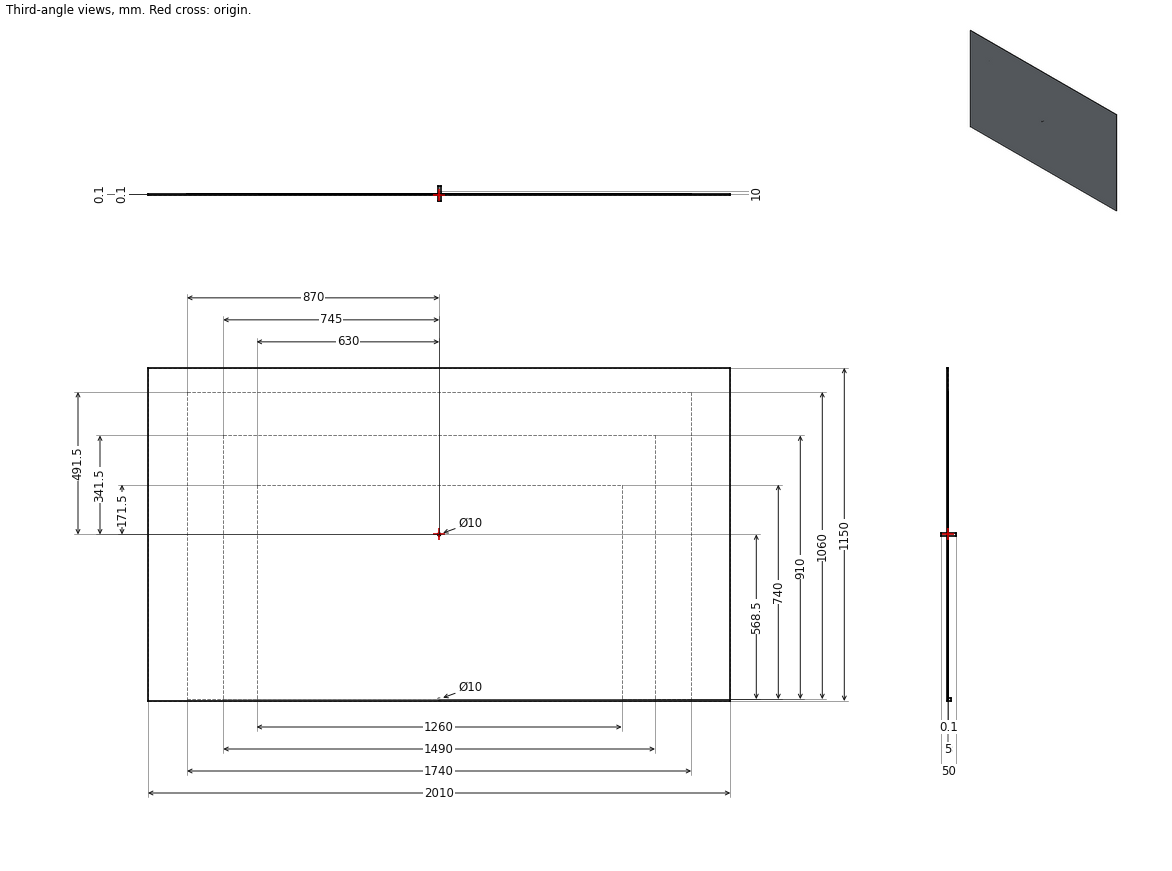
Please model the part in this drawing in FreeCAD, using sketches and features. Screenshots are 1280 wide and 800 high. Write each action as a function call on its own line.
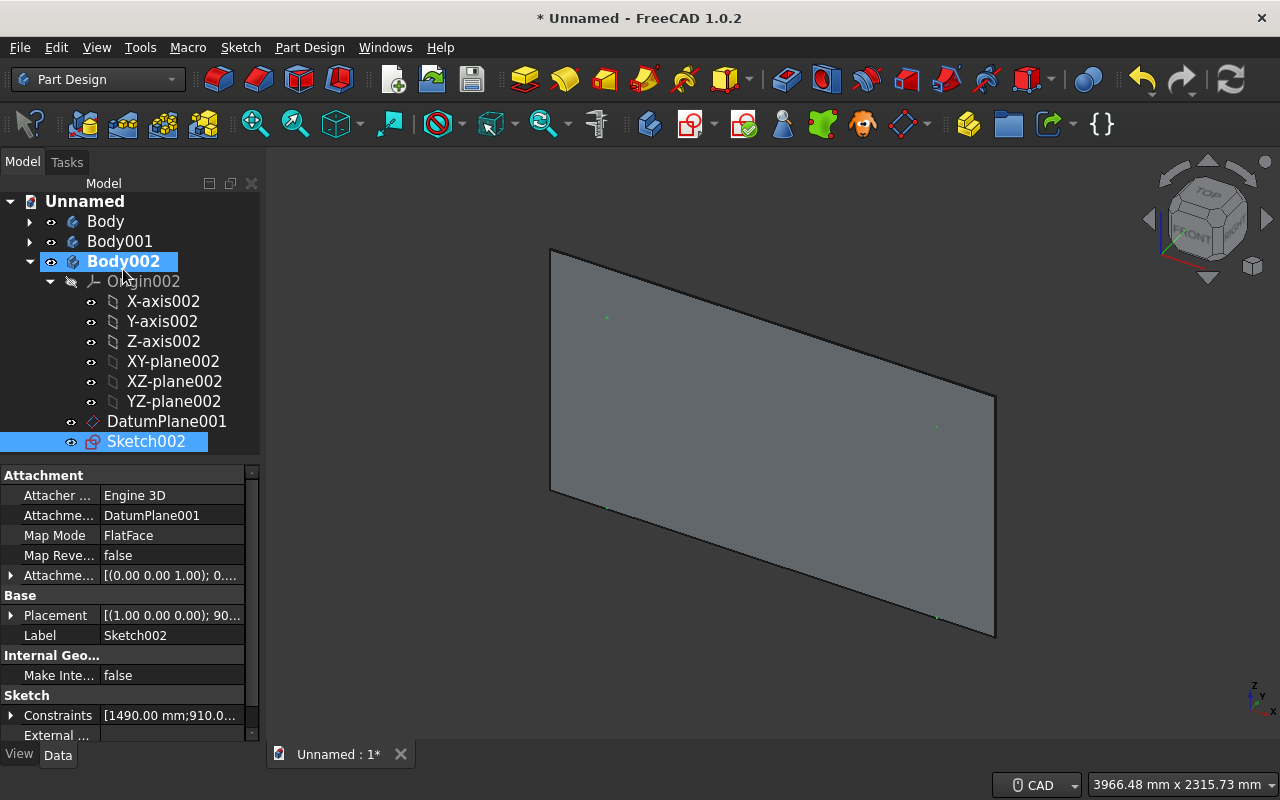
click(526, 80)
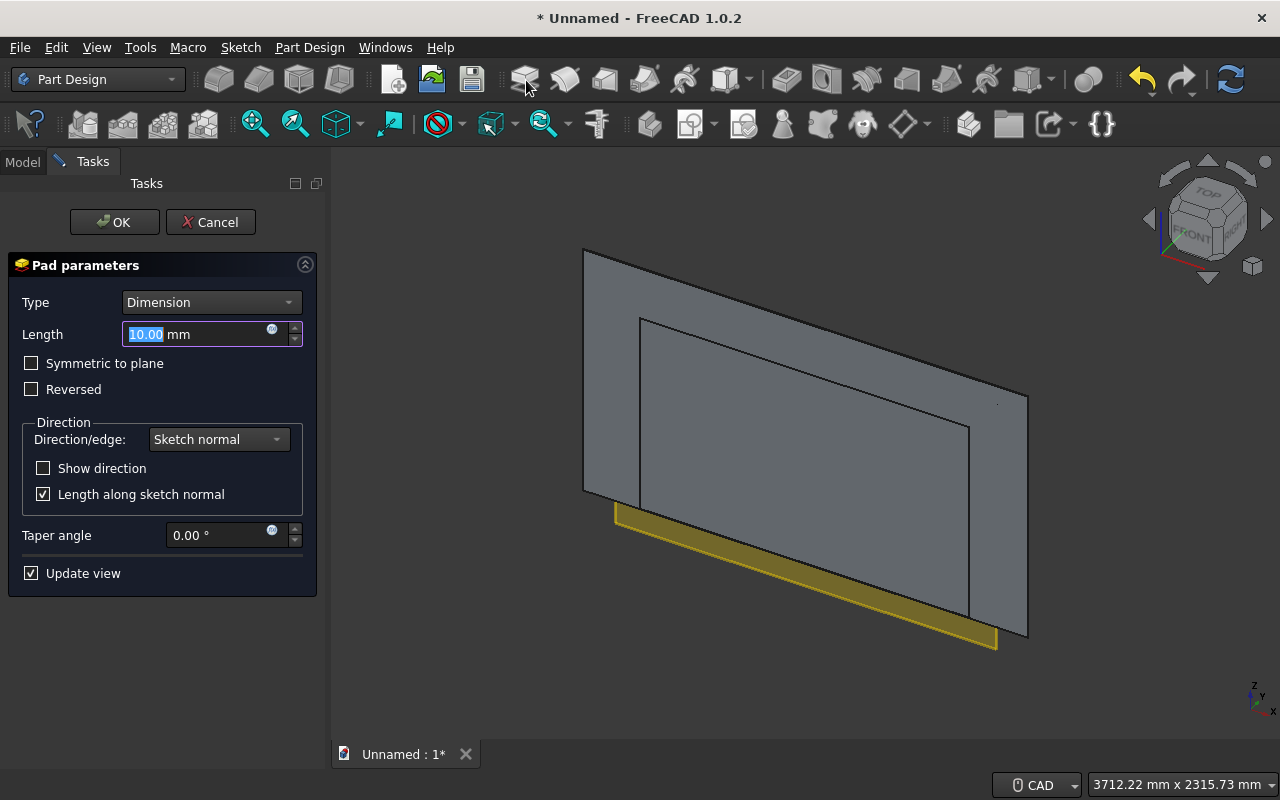
text(0.1)
key(Tab)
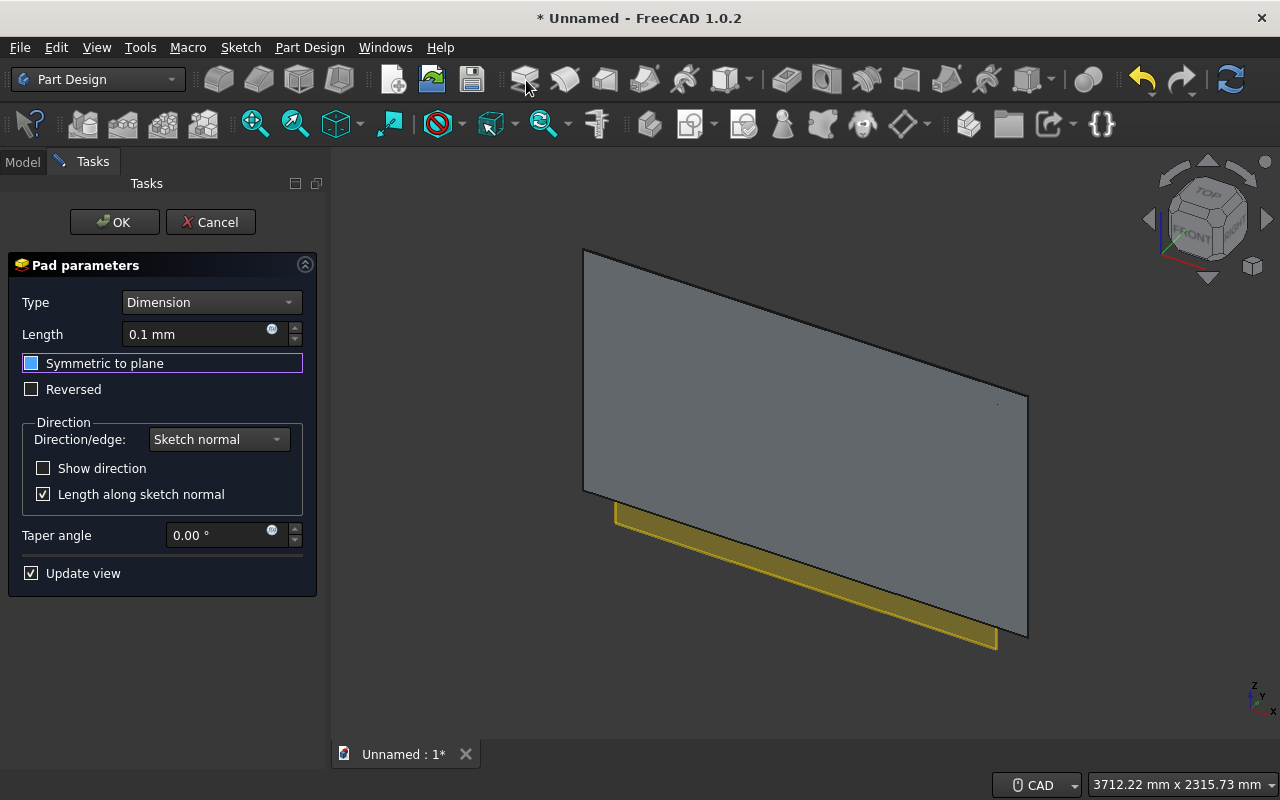
click(30, 389)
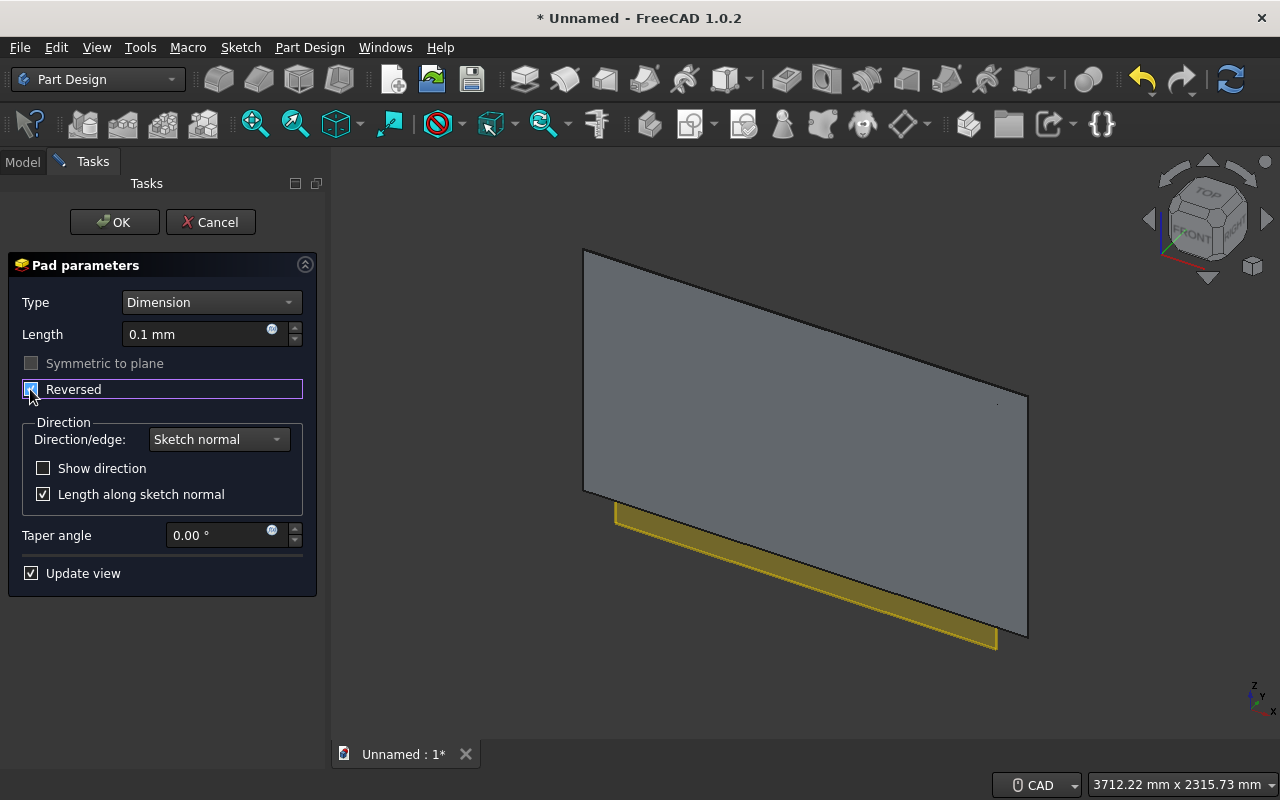
click(115, 222)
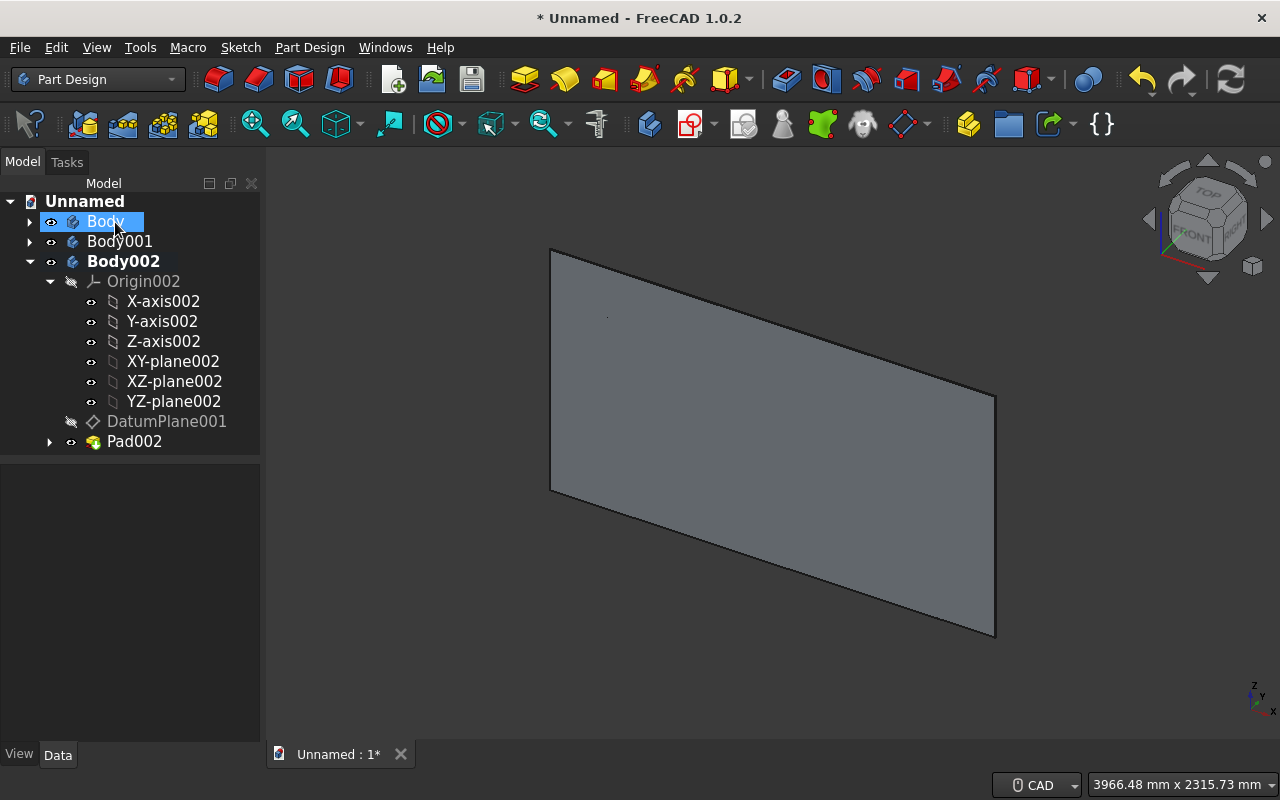
click(650, 124)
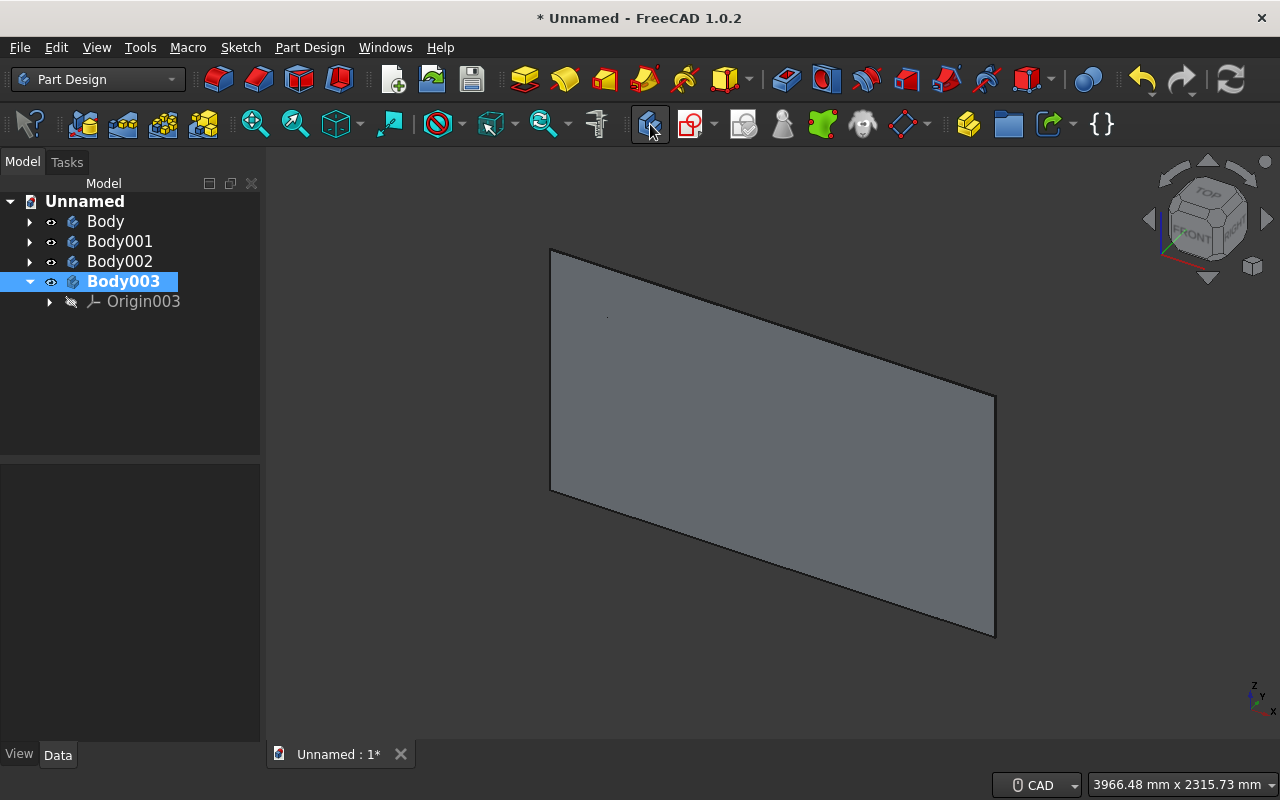
click(50, 302)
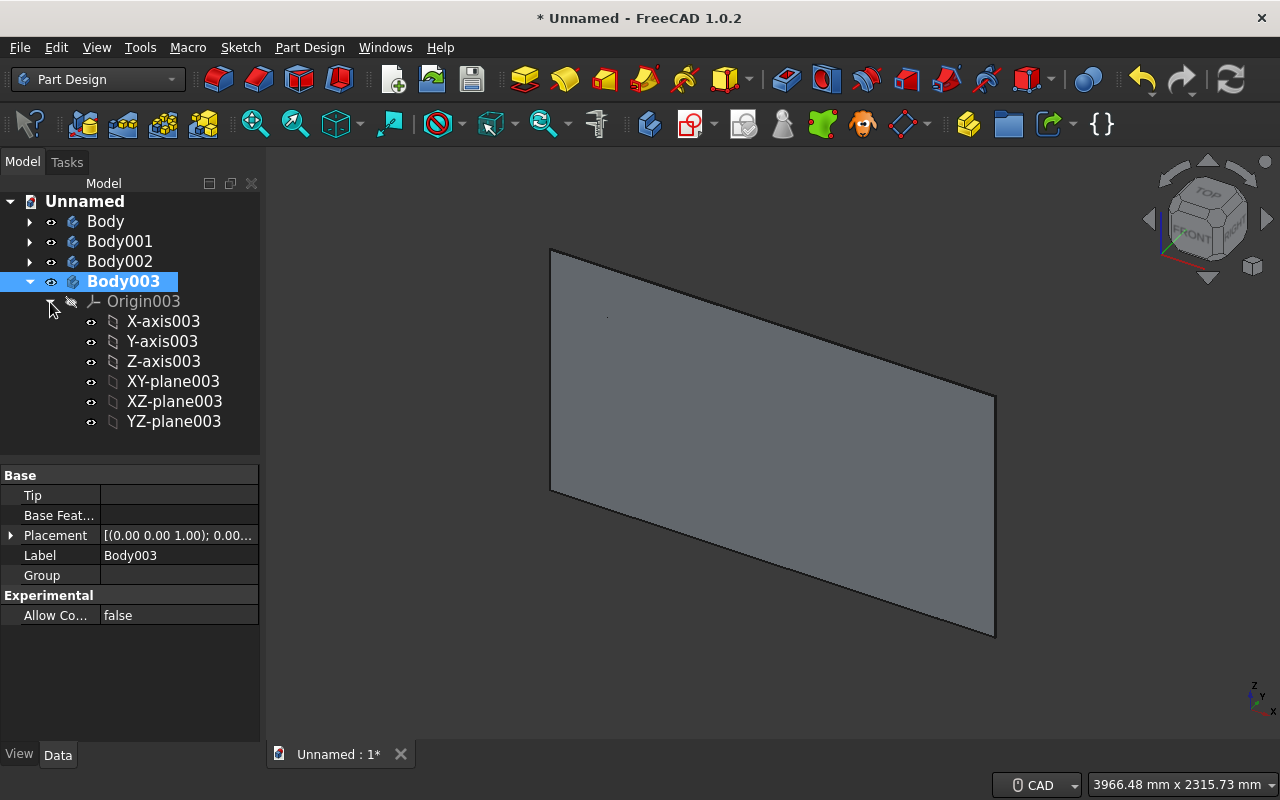
click(136, 402)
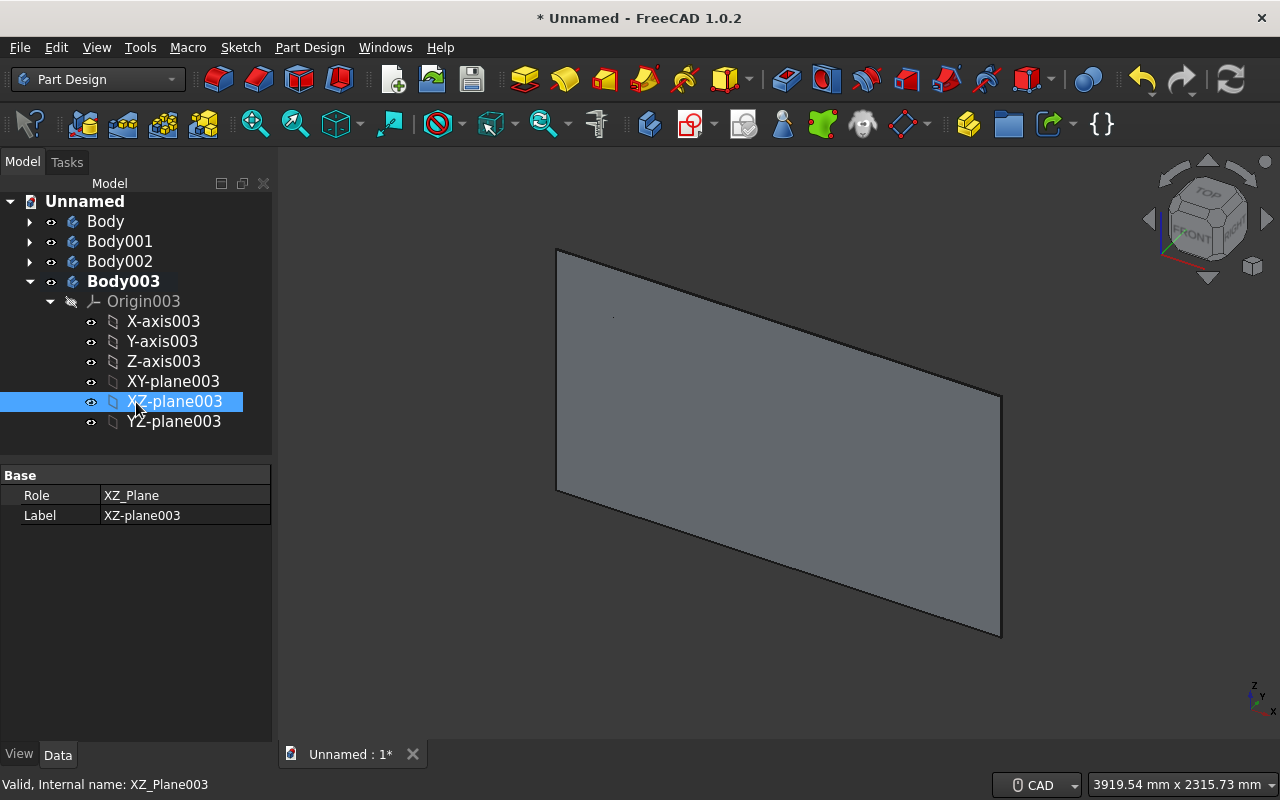
click(904, 124)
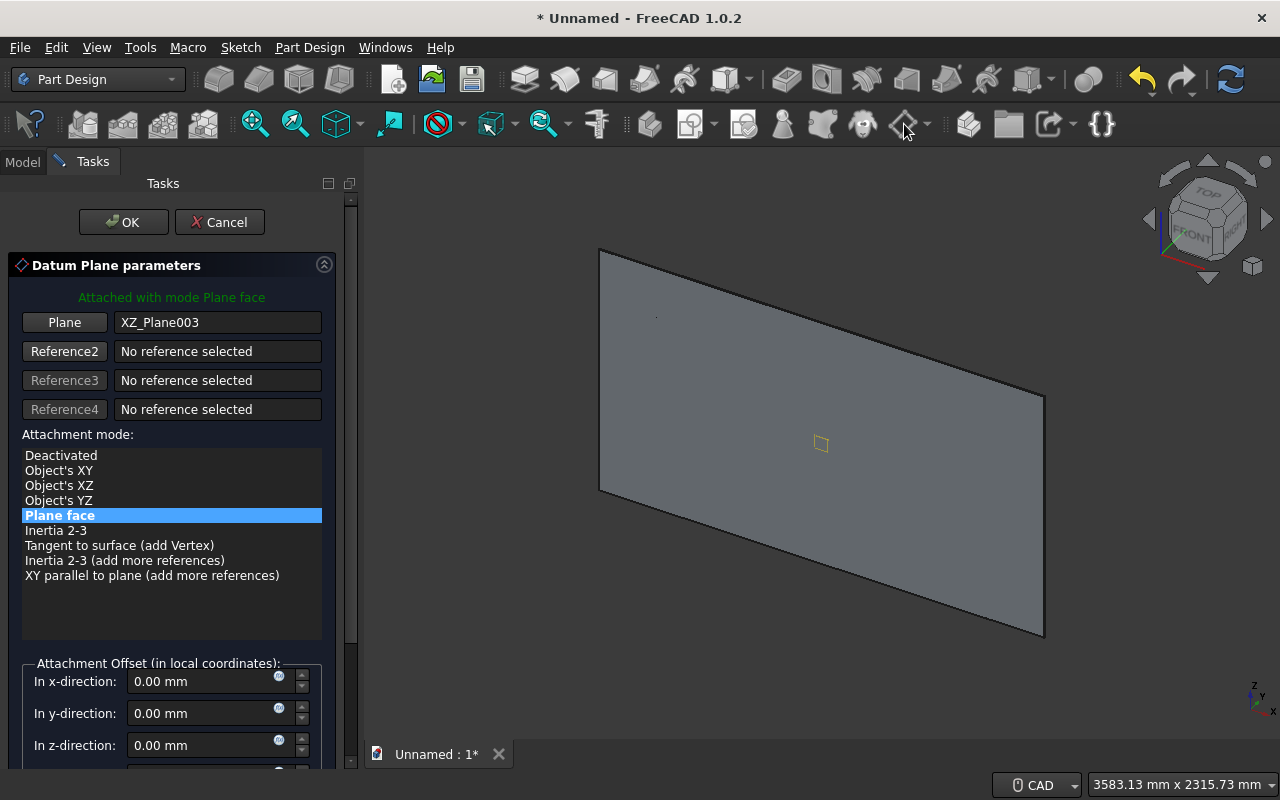
triple_click(210, 745)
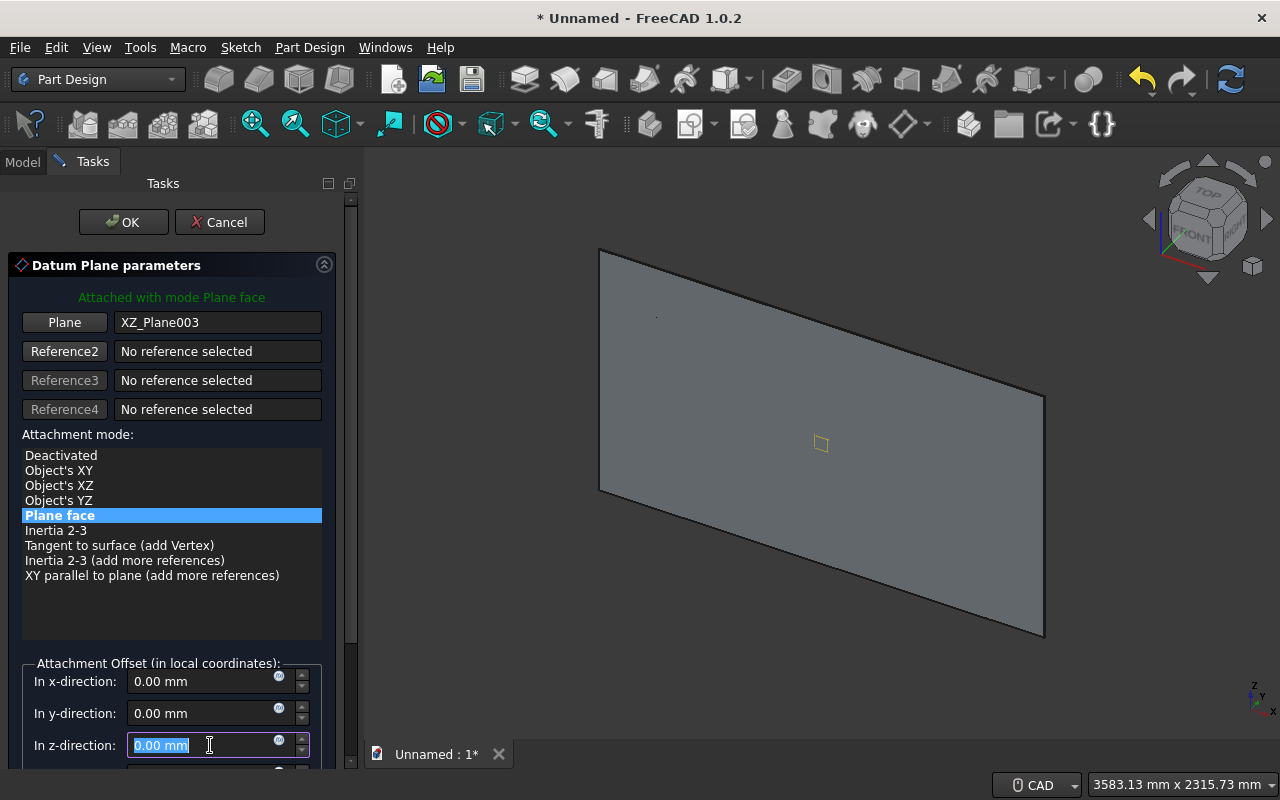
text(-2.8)
key(Tab)